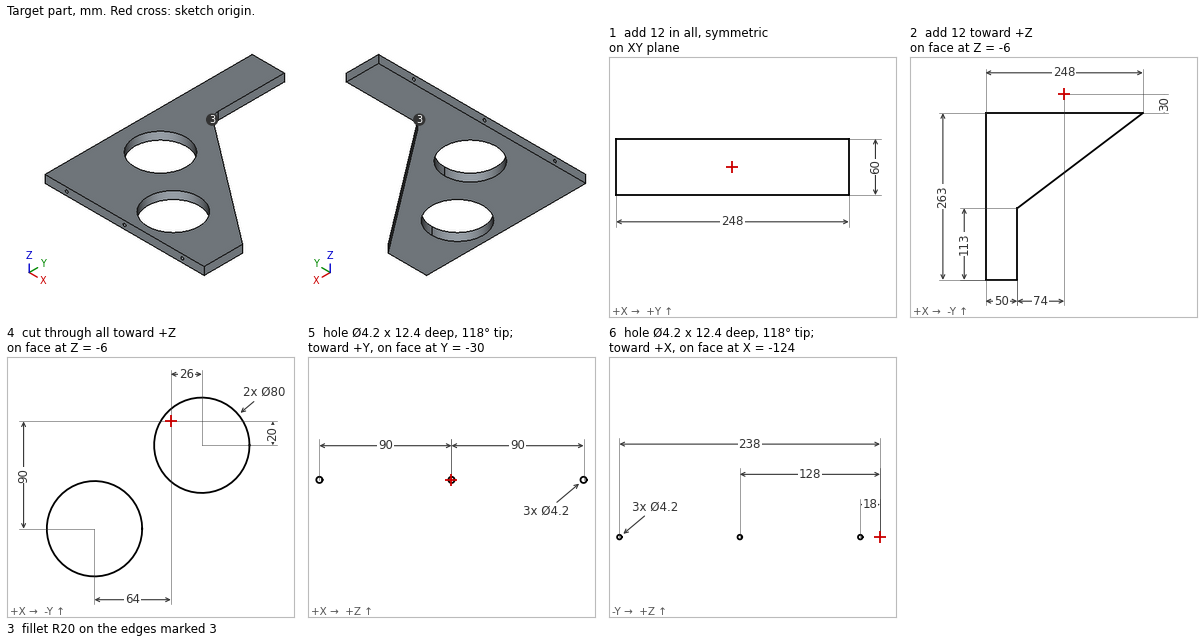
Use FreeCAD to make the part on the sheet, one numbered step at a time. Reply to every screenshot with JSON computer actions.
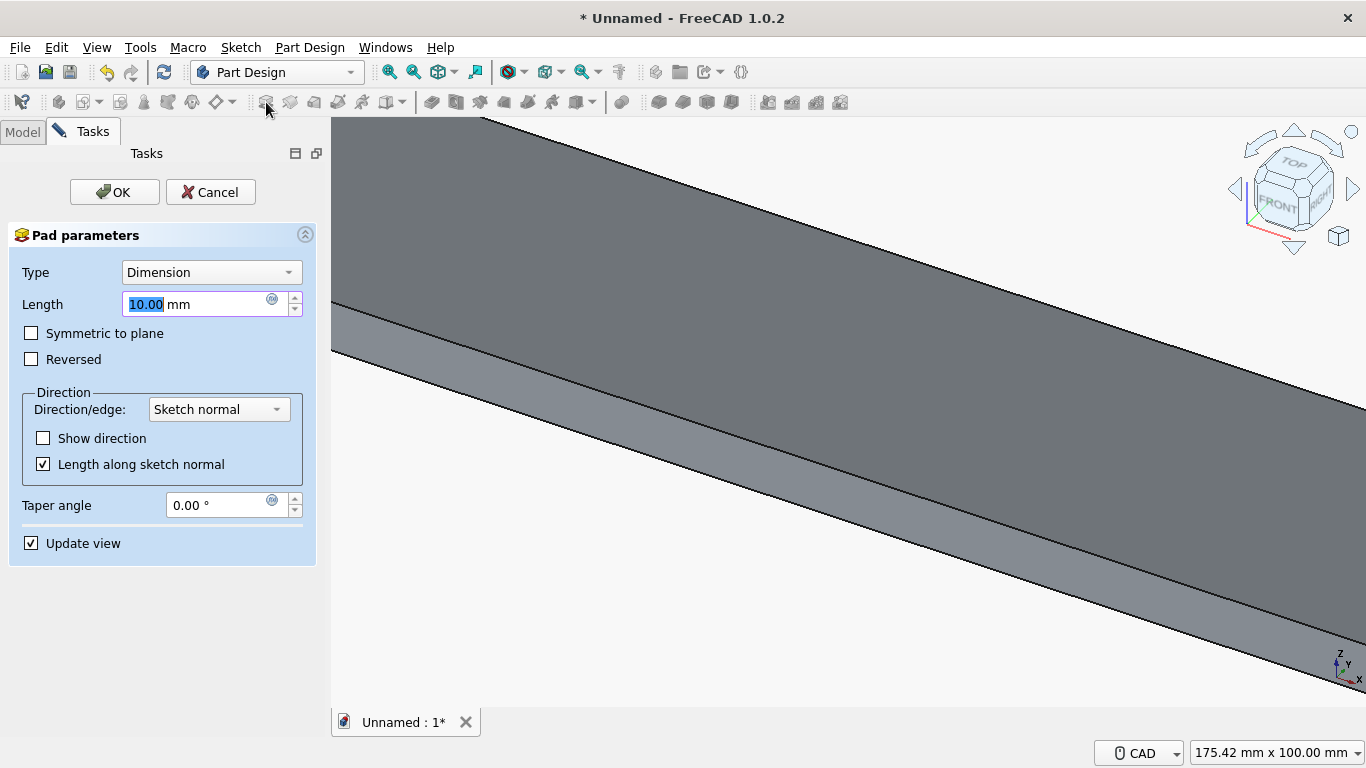
{"action": "type", "text": "12"}
{"action": "key", "text": "Tab"}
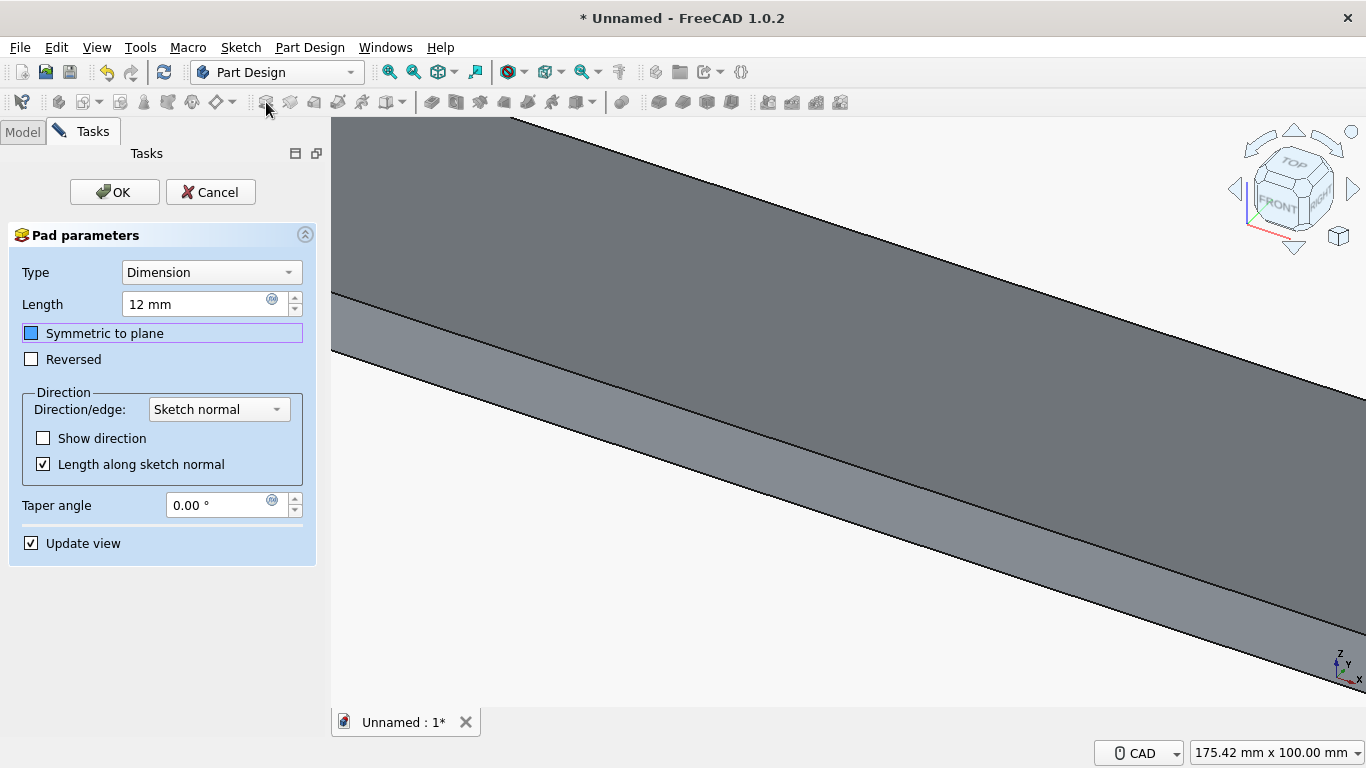
{"action": "left_click", "coordinate": [30, 333]}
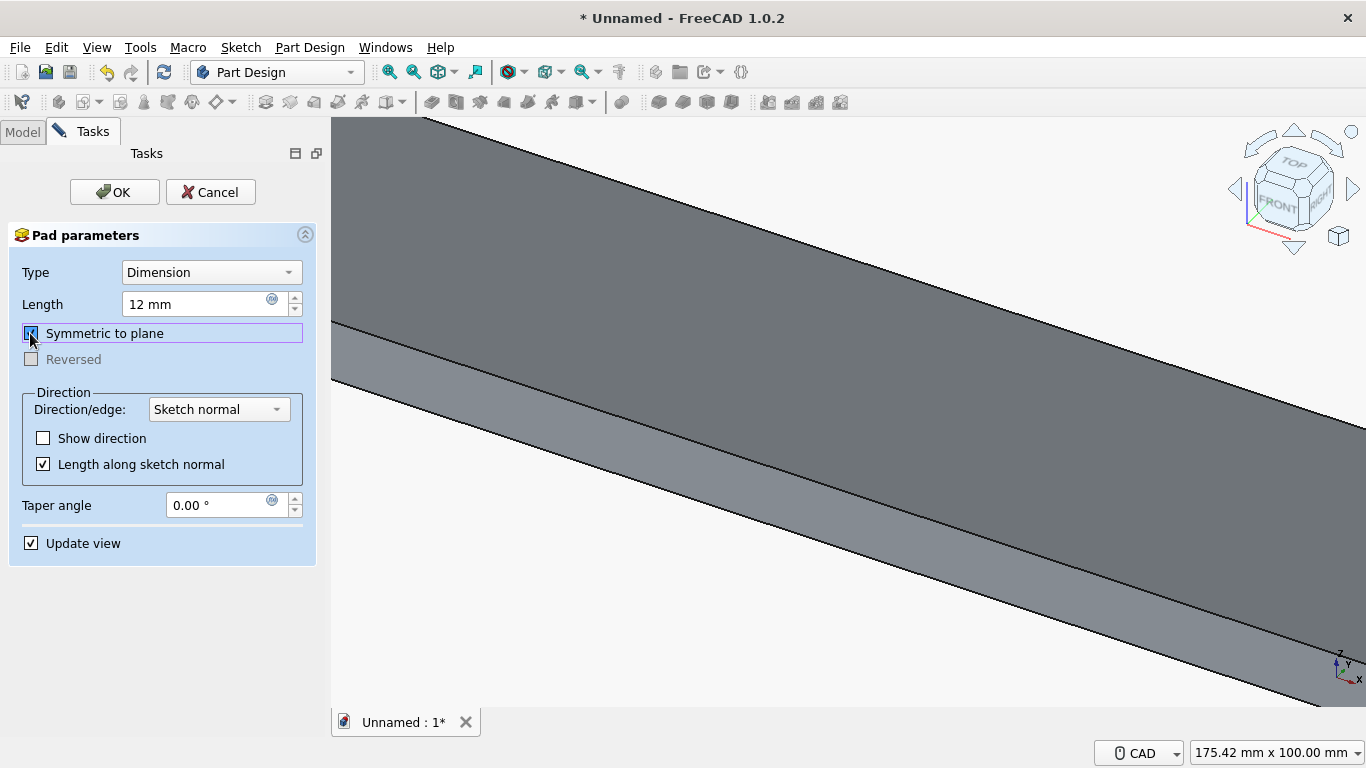
{"action": "left_click", "coordinate": [115, 192]}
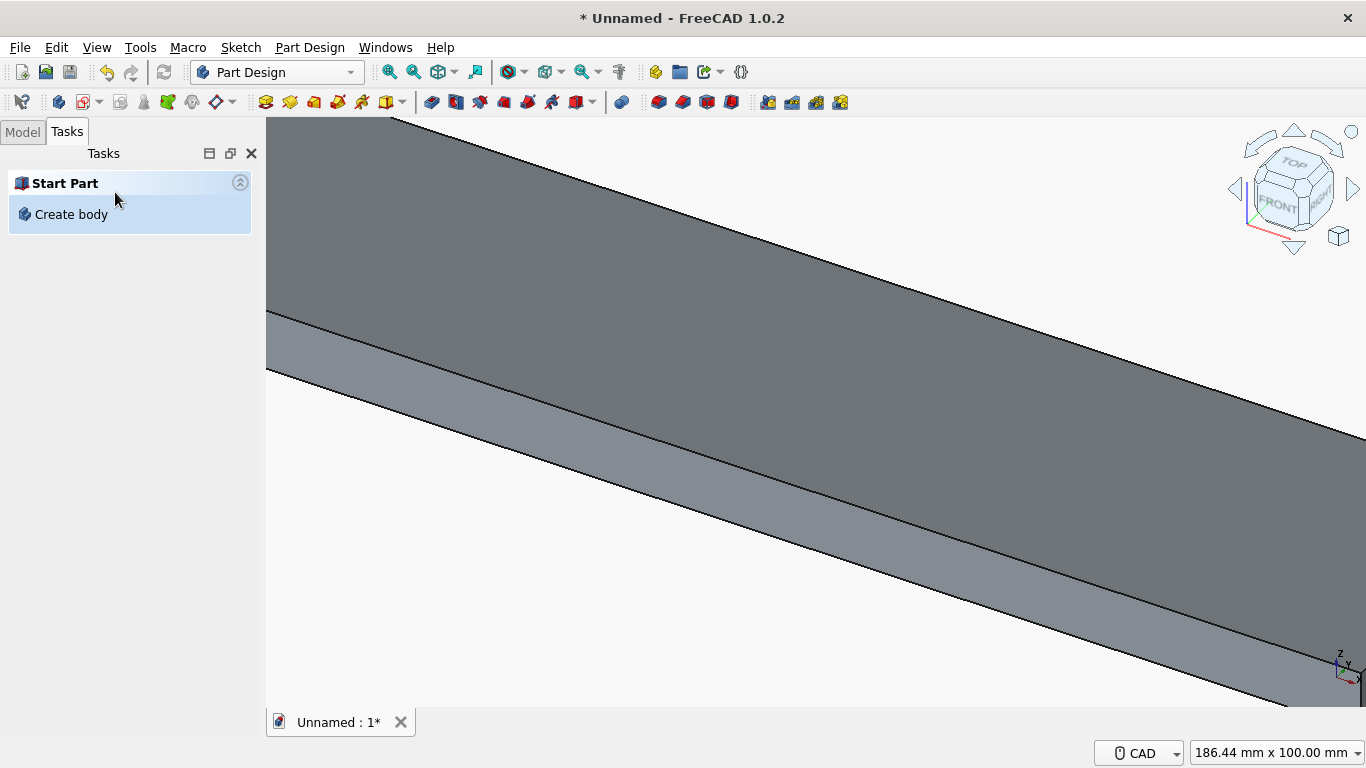
{"action": "key", "text": "v f"}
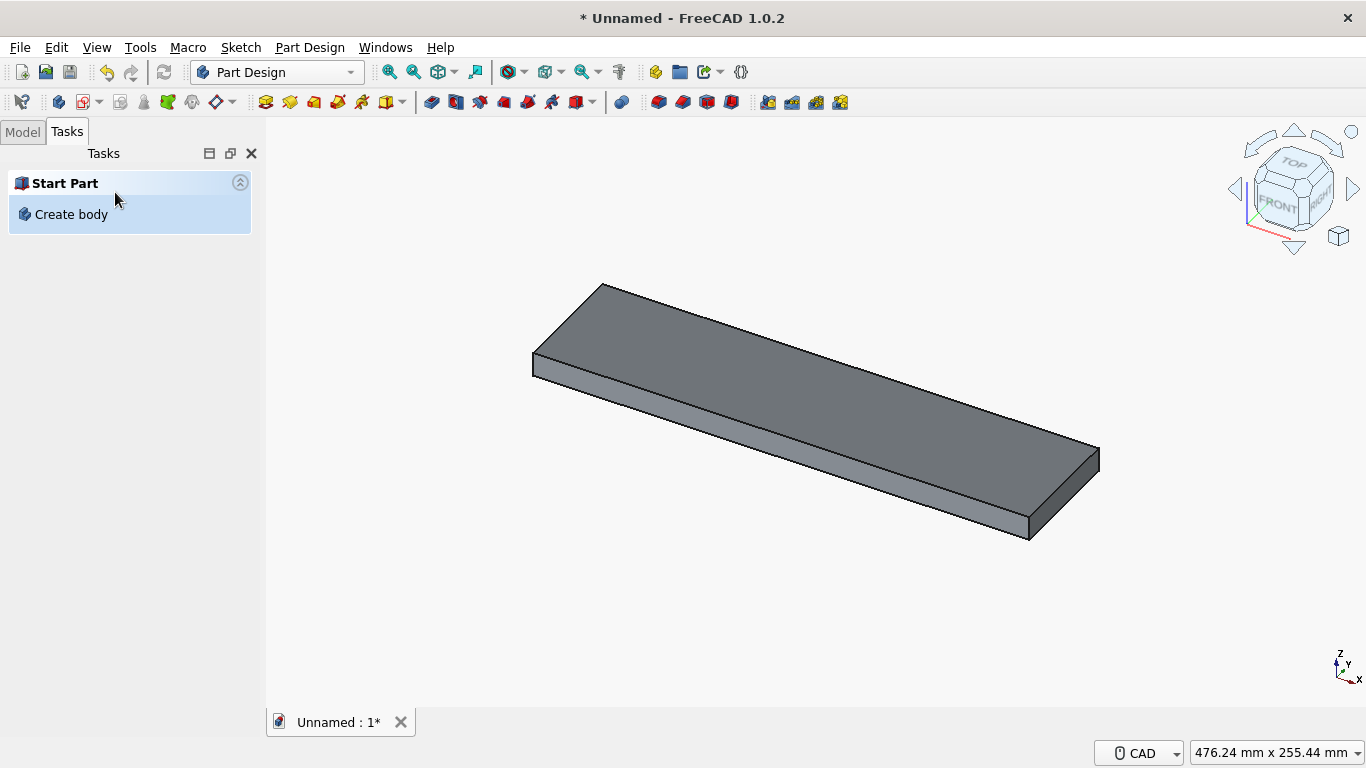
{"action": "key", "text": "5"}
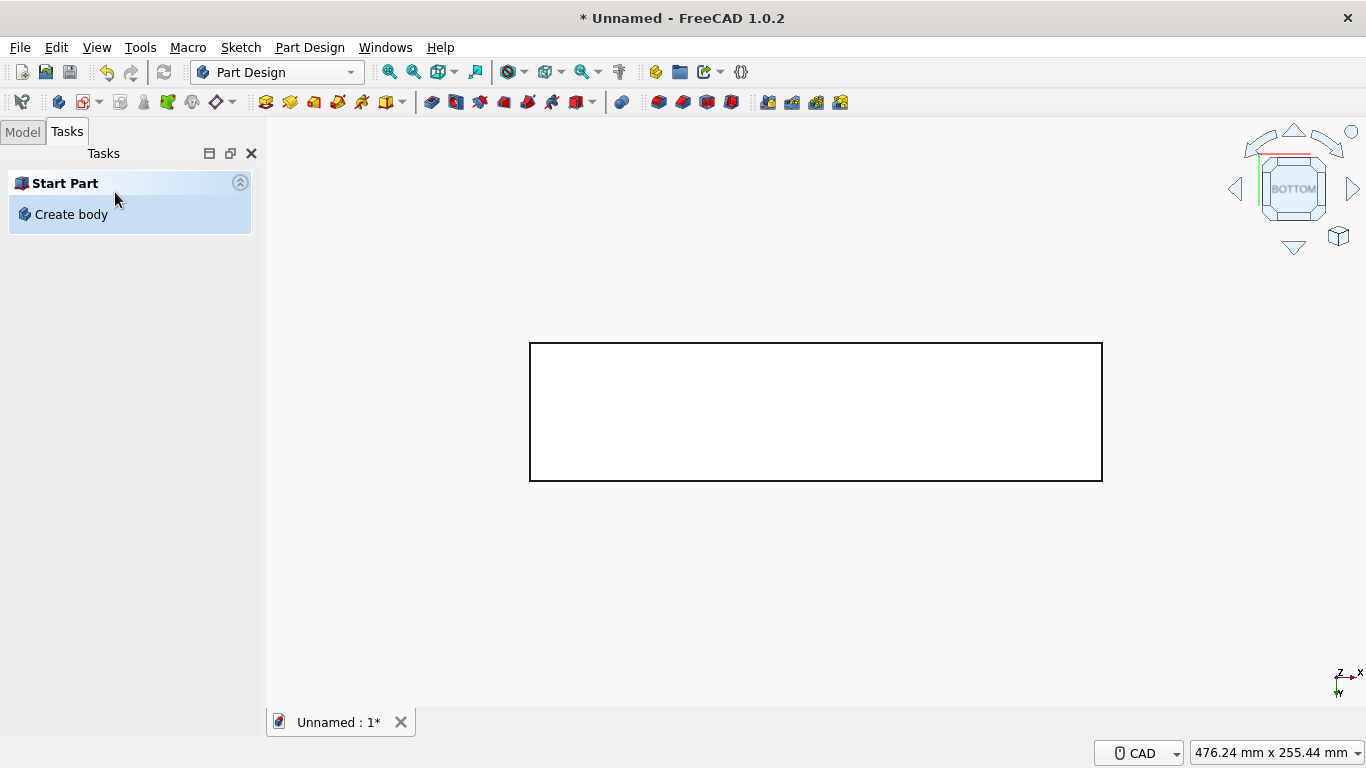
{"action": "left_click", "coordinate": [980, 411]}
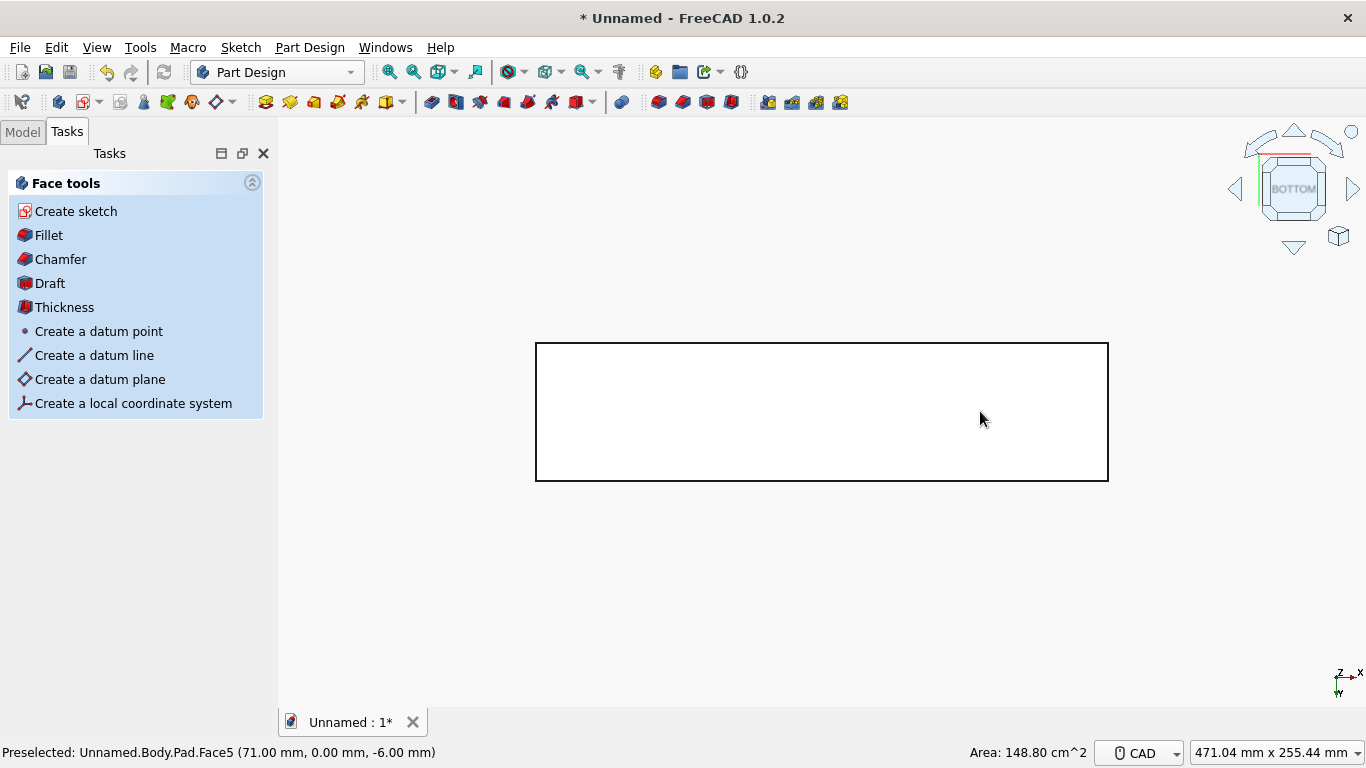
{"action": "left_click", "coordinate": [84, 102]}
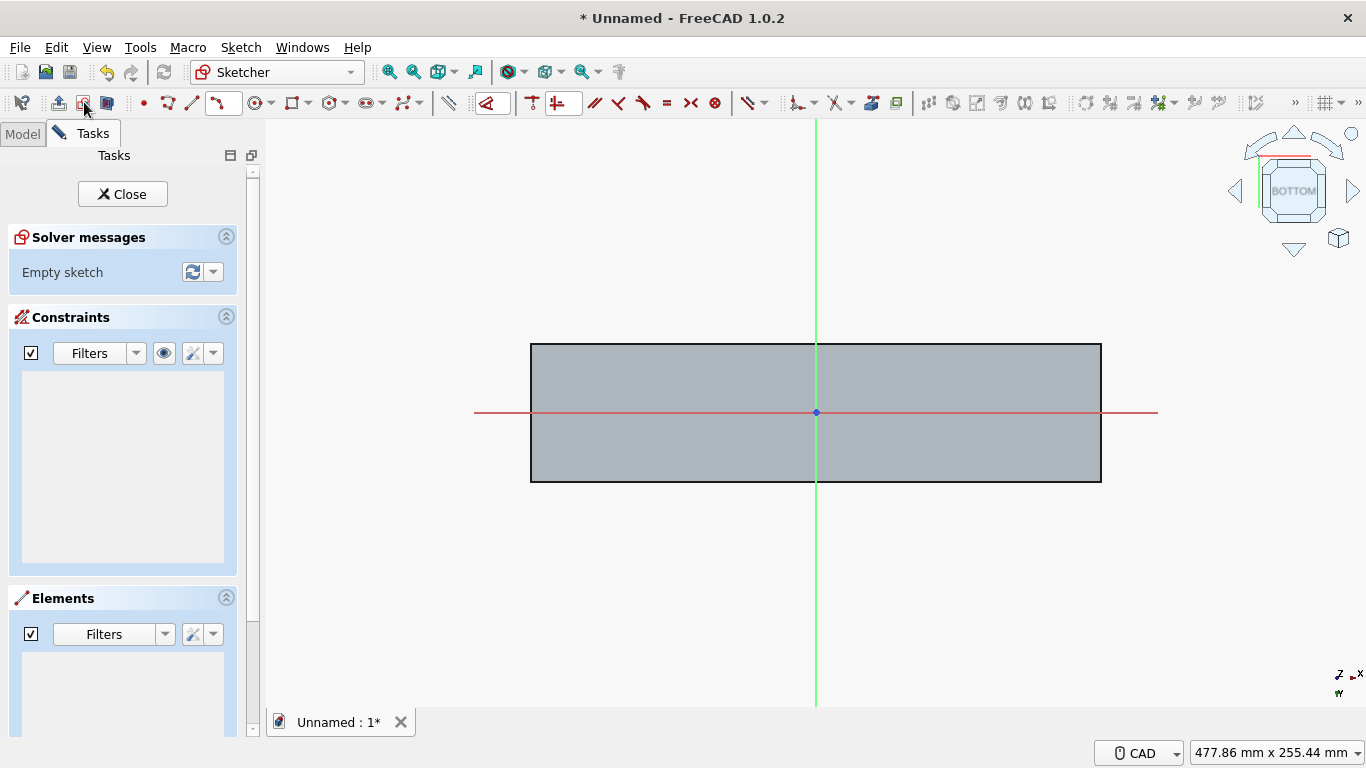
{"action": "scroll", "coordinate": [692, 147], "scroll_direction": "down", "scroll_amount": 4}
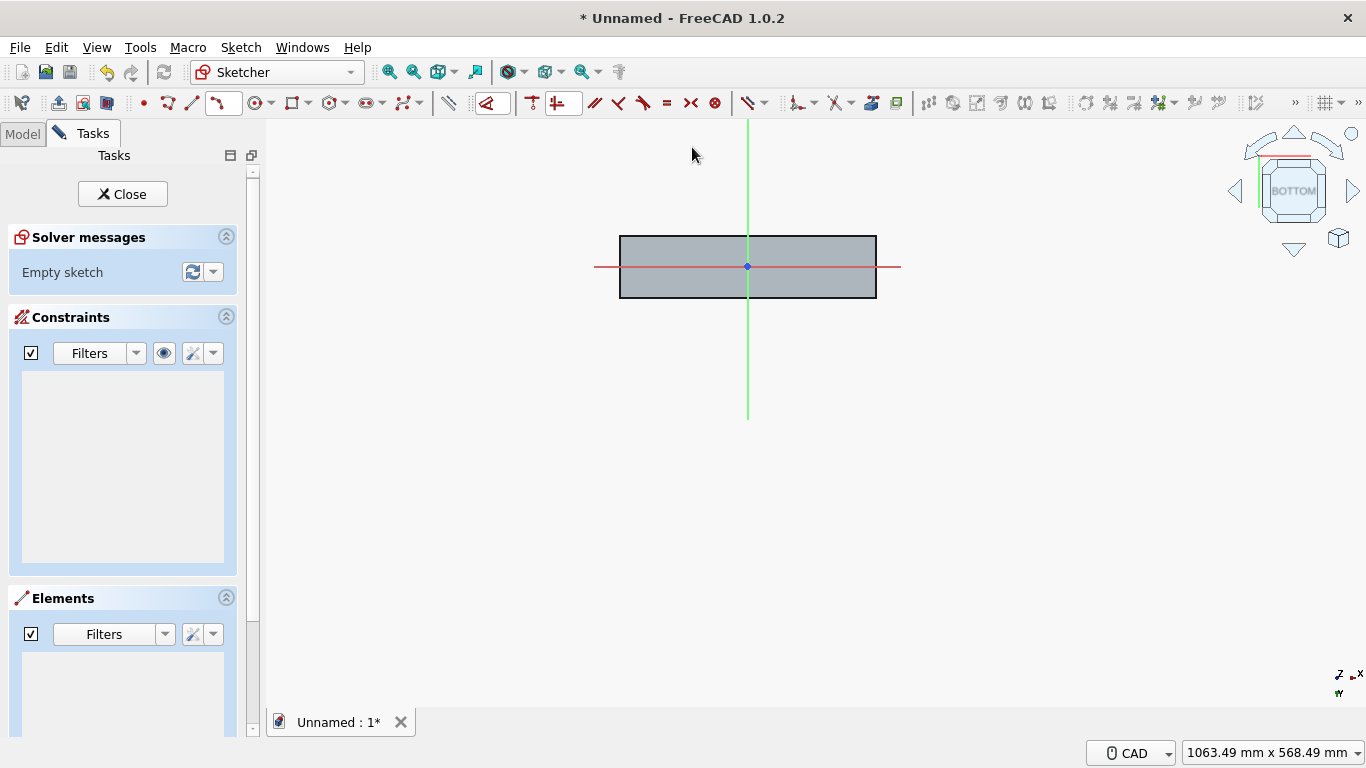
{"action": "key", "text": "g m"}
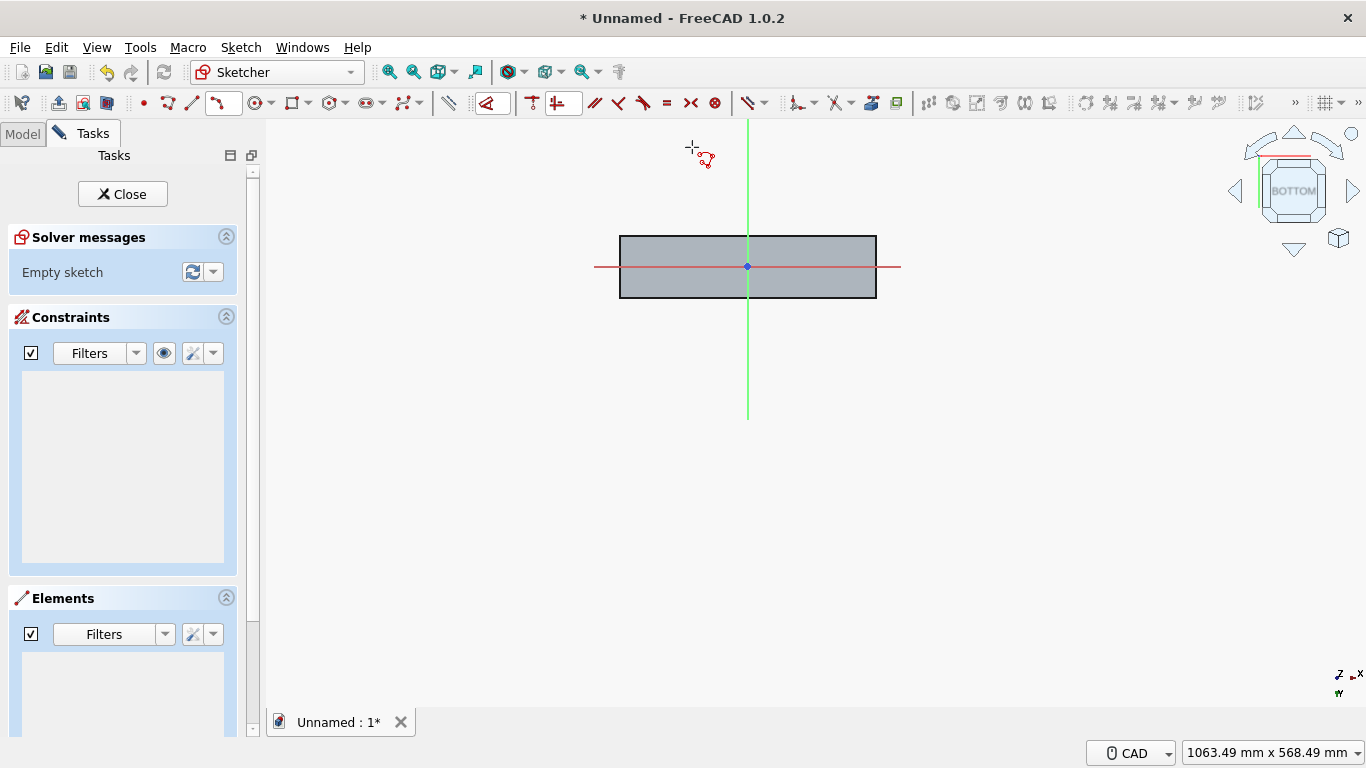
{"action": "left_click", "coordinate": [876, 298]}
{"action": "left_click", "coordinate": [620, 298]}
{"action": "left_click", "coordinate": [620, 570]}
{"action": "left_click", "coordinate": [671, 570]}
{"action": "left_click", "coordinate": [671, 453]}
{"action": "left_click", "coordinate": [876, 299]}
{"action": "key", "text": "Escape"}
{"action": "key", "text": "Escape"}